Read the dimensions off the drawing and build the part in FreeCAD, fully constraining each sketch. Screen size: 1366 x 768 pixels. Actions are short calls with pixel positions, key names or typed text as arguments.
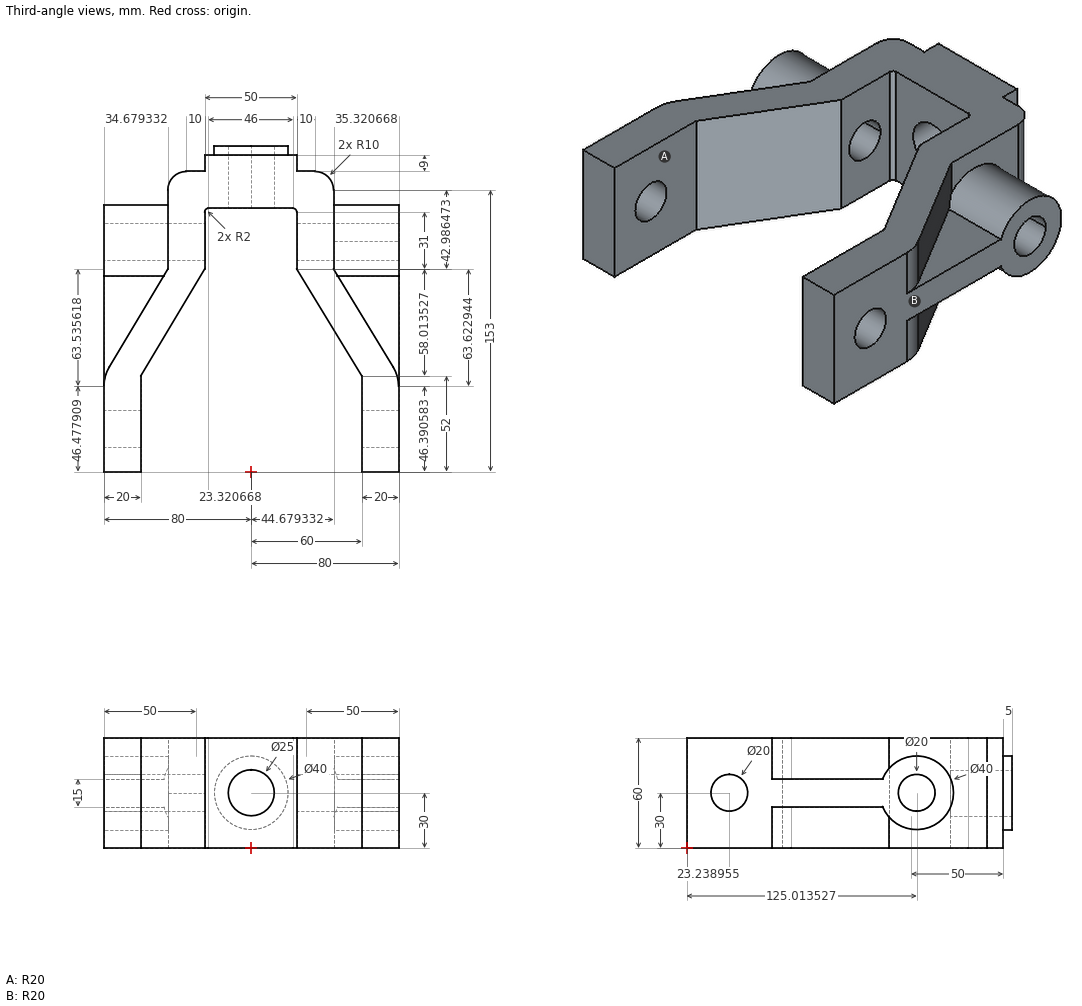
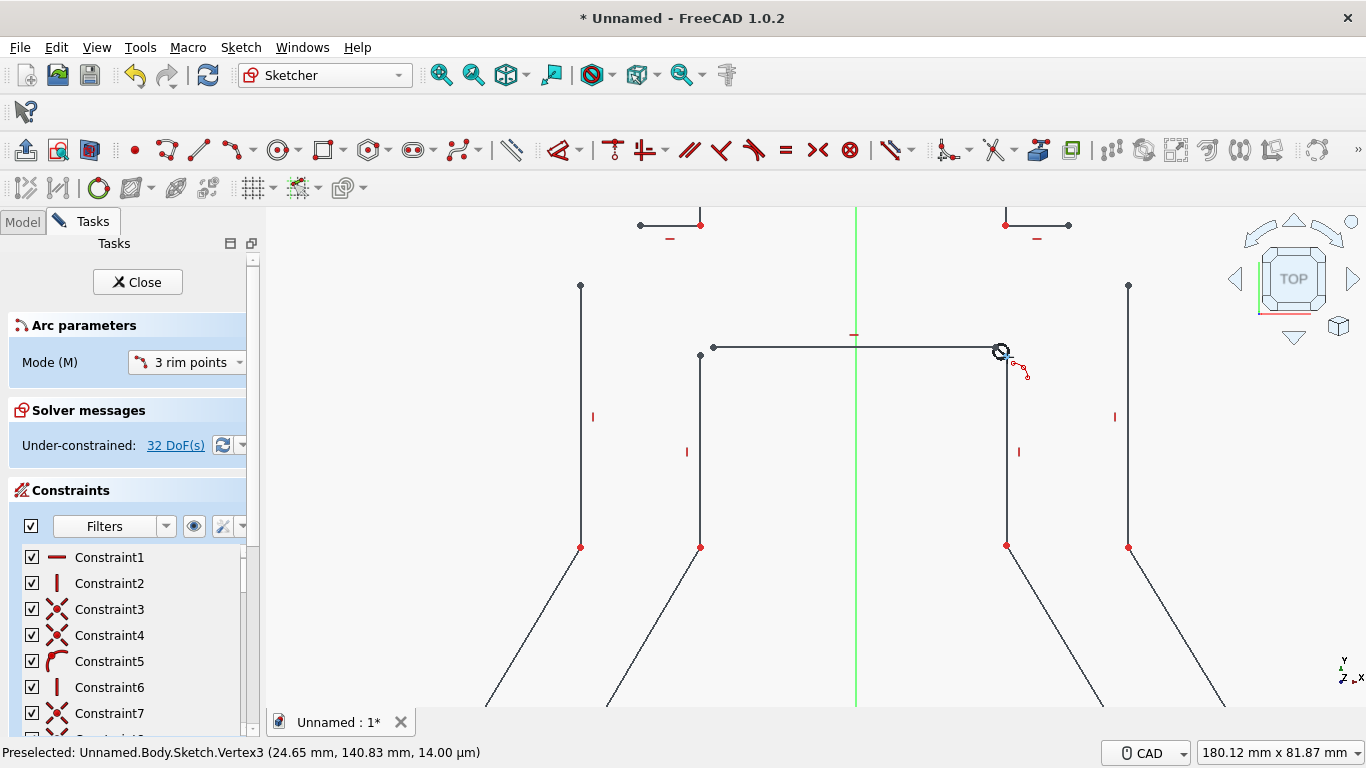
scroll(1003, 347, up, 8)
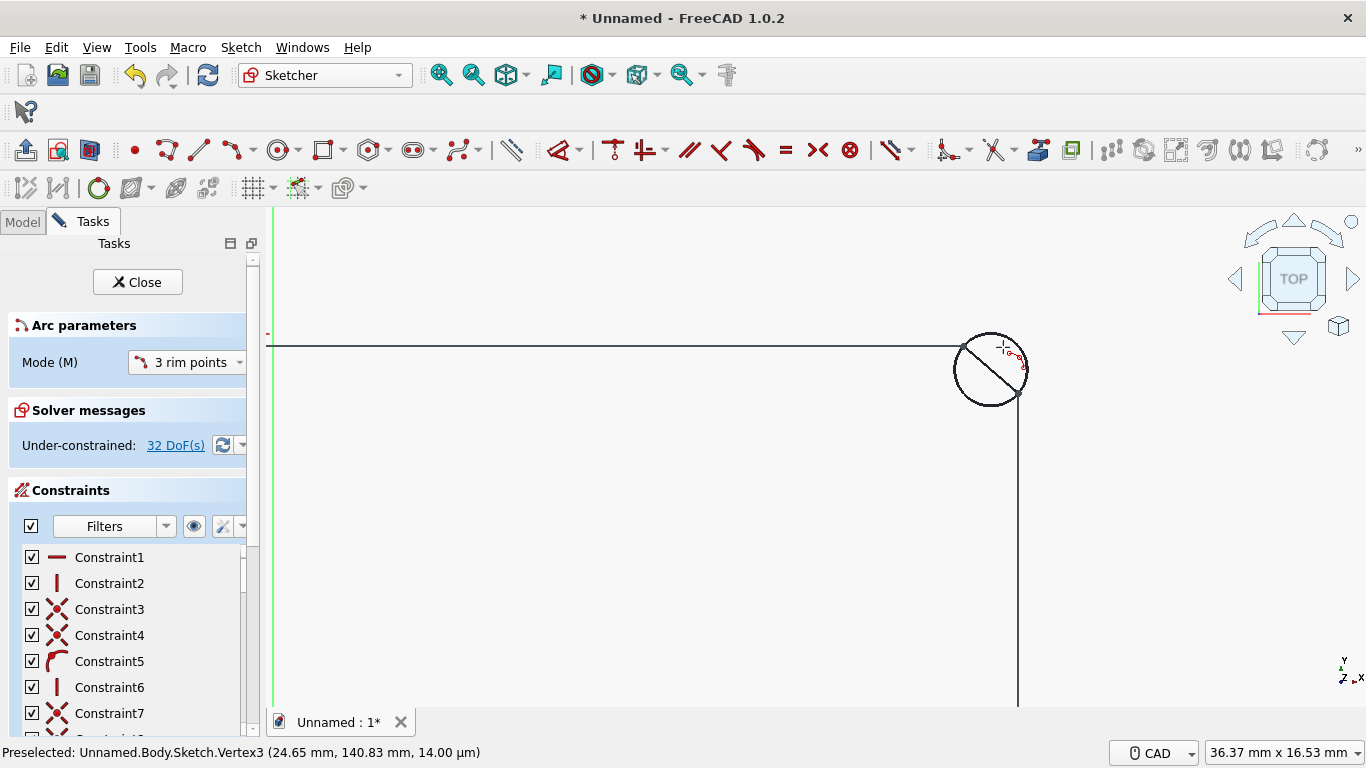
click(1001, 345)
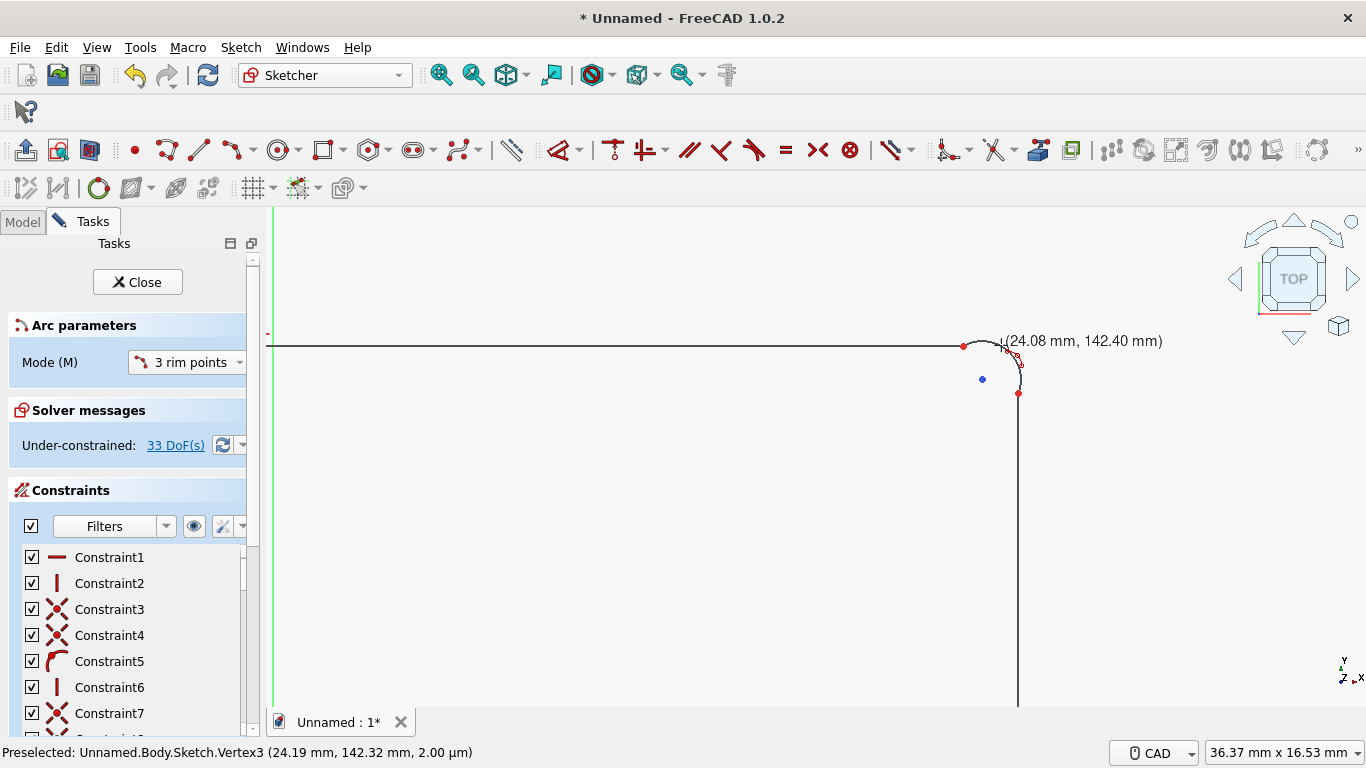
scroll(778, 354, down, 14)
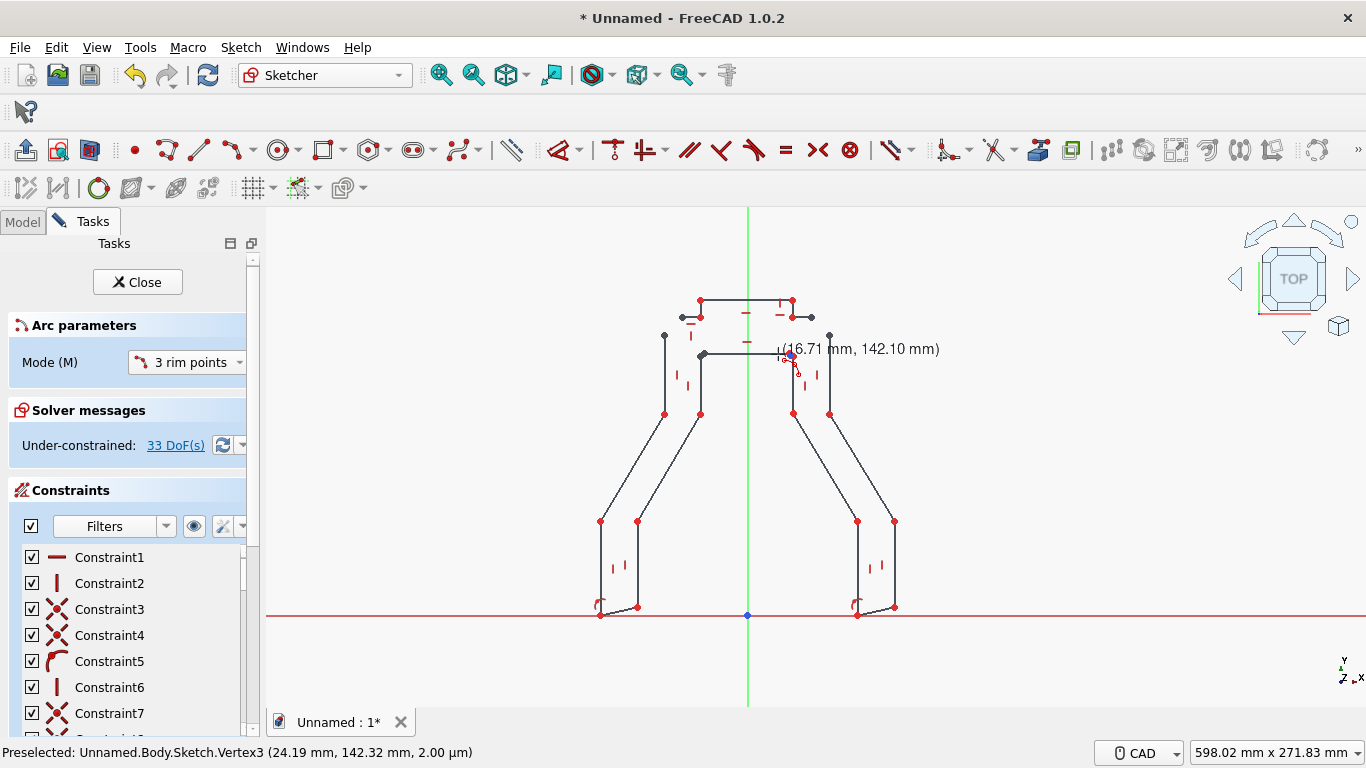
click(830, 335)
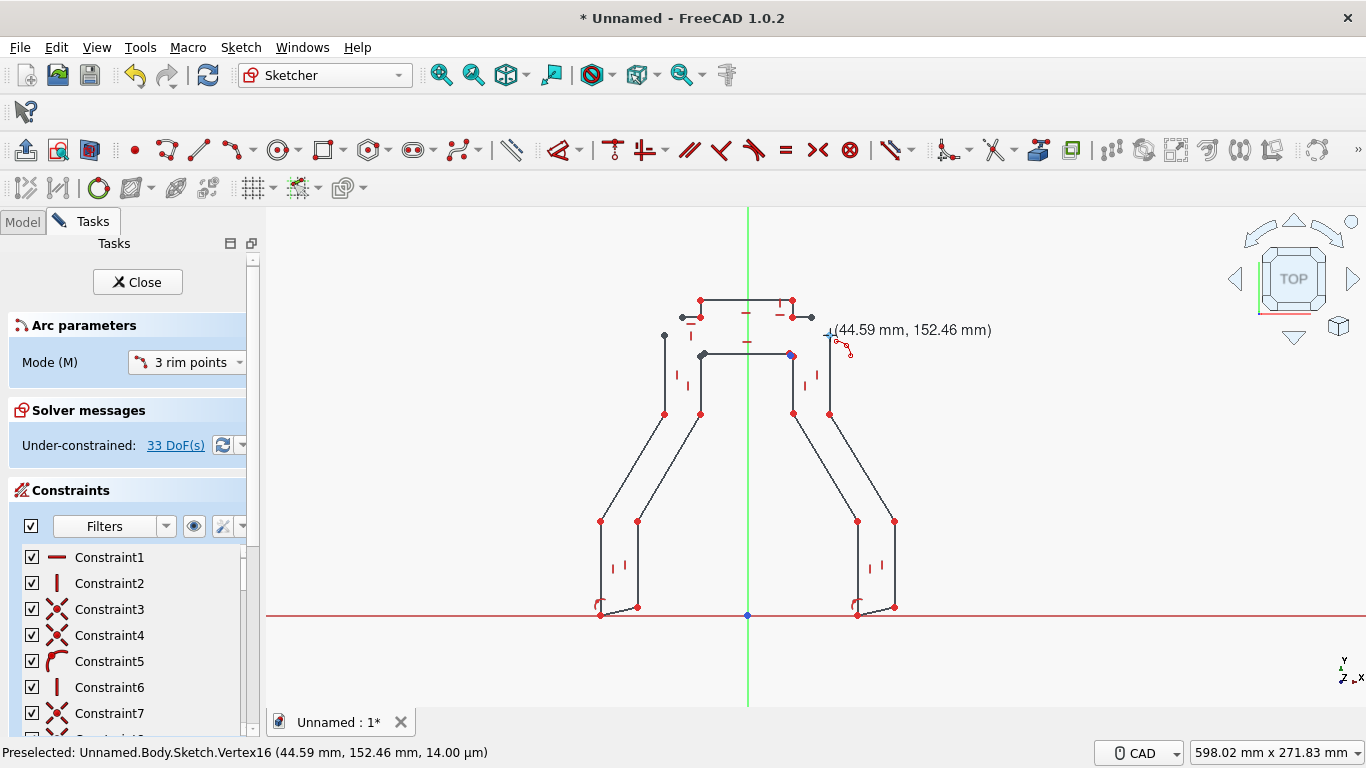
scroll(811, 316, up, 3)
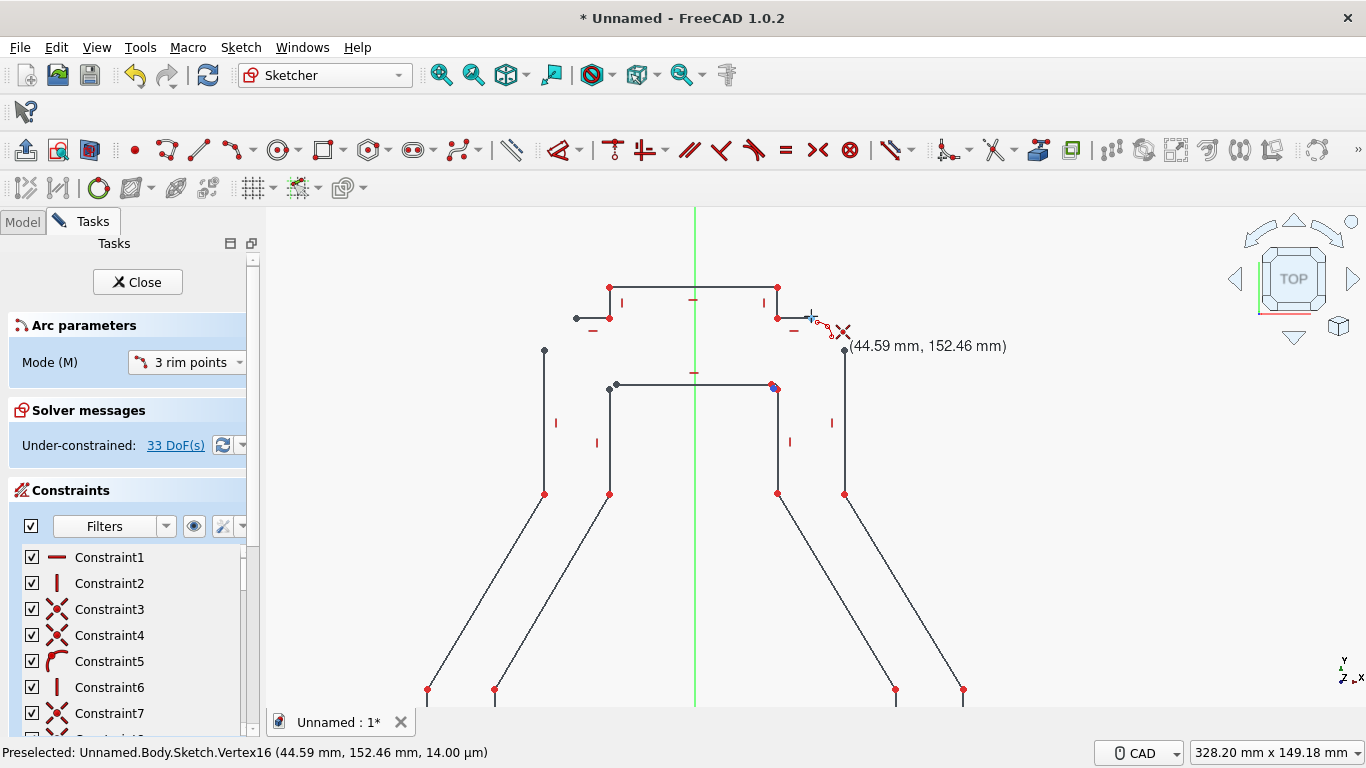
click(812, 318)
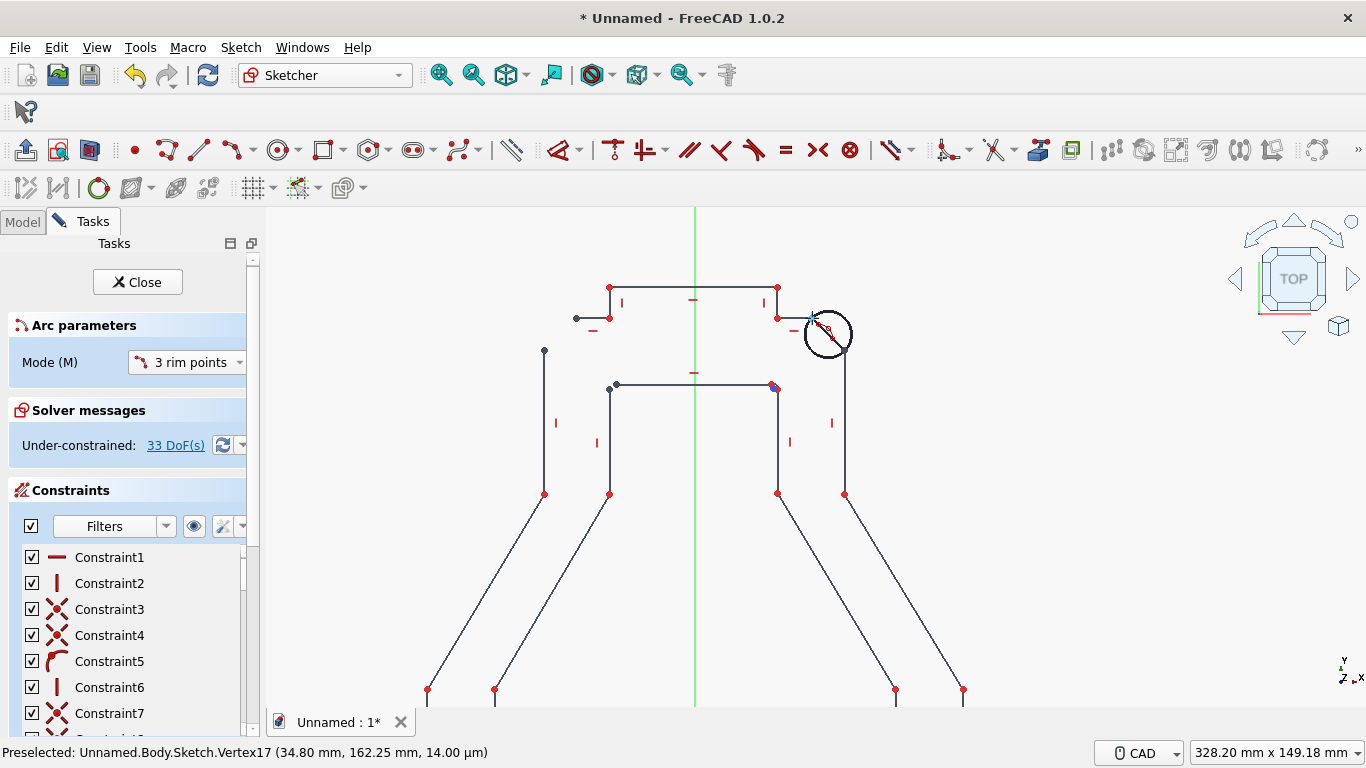
scroll(835, 325, up, 3)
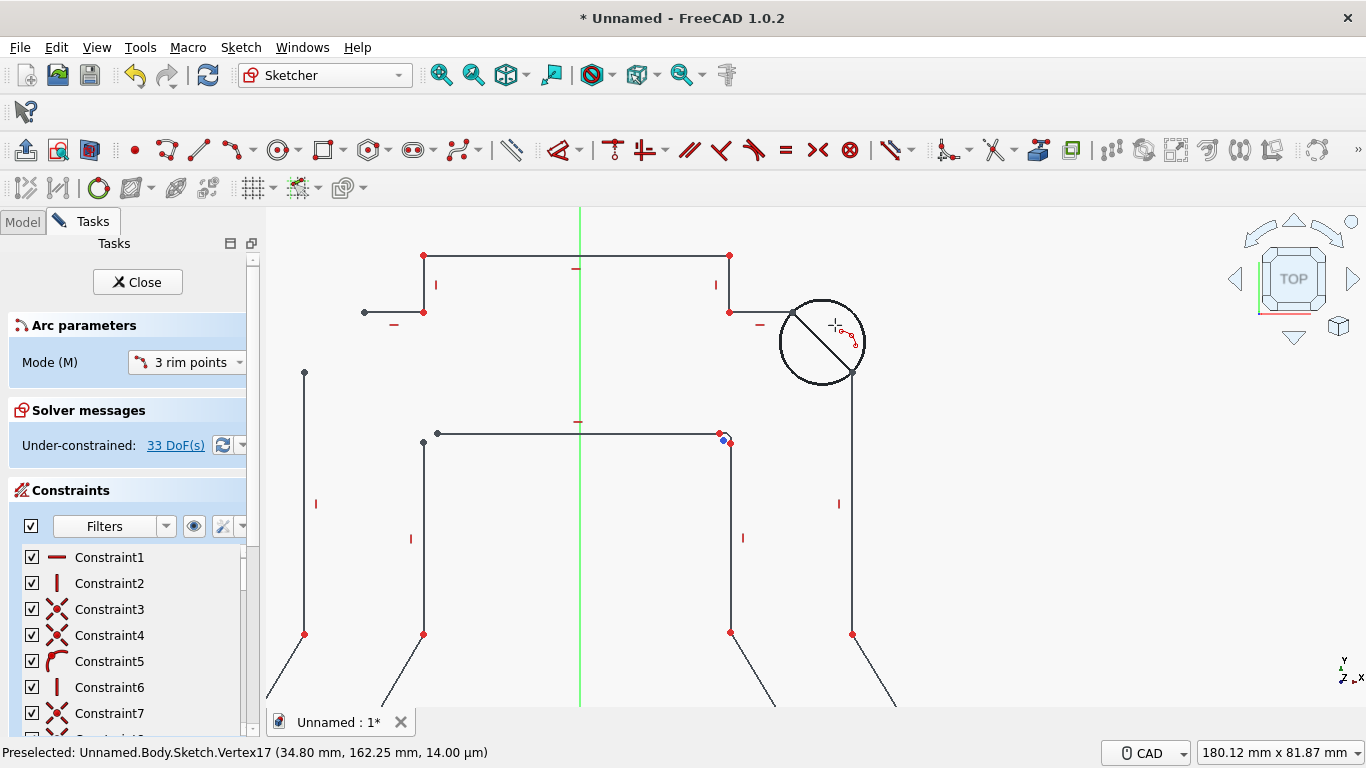
click(835, 326)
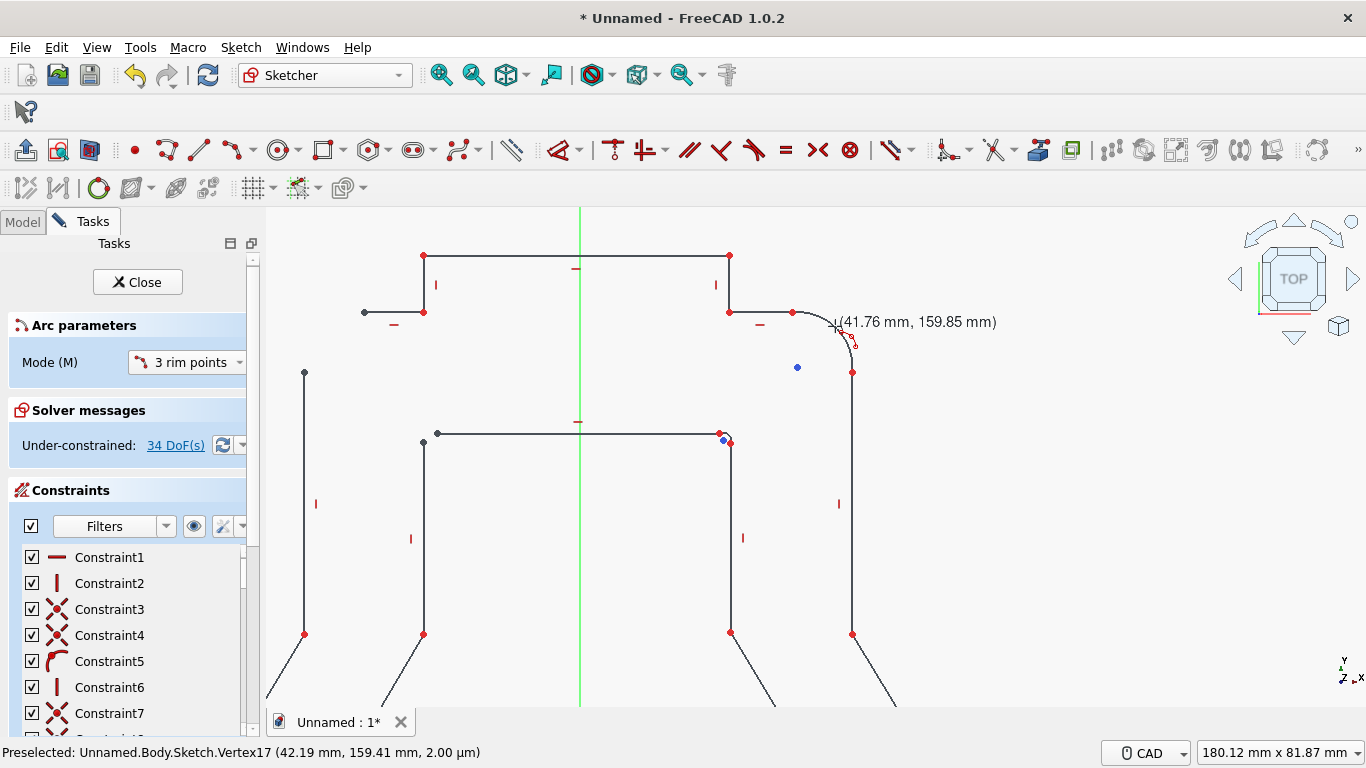
click(364, 312)
click(304, 372)
click(321, 326)